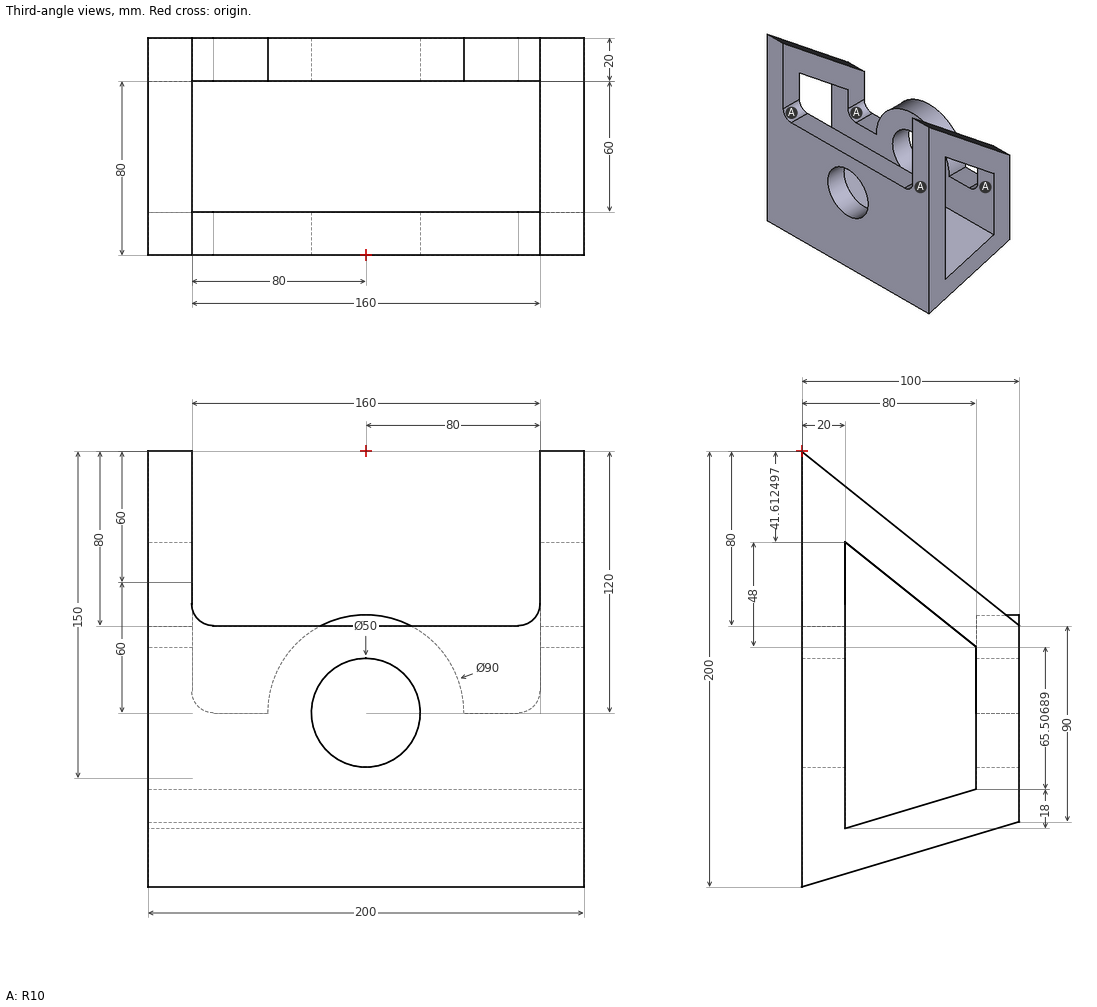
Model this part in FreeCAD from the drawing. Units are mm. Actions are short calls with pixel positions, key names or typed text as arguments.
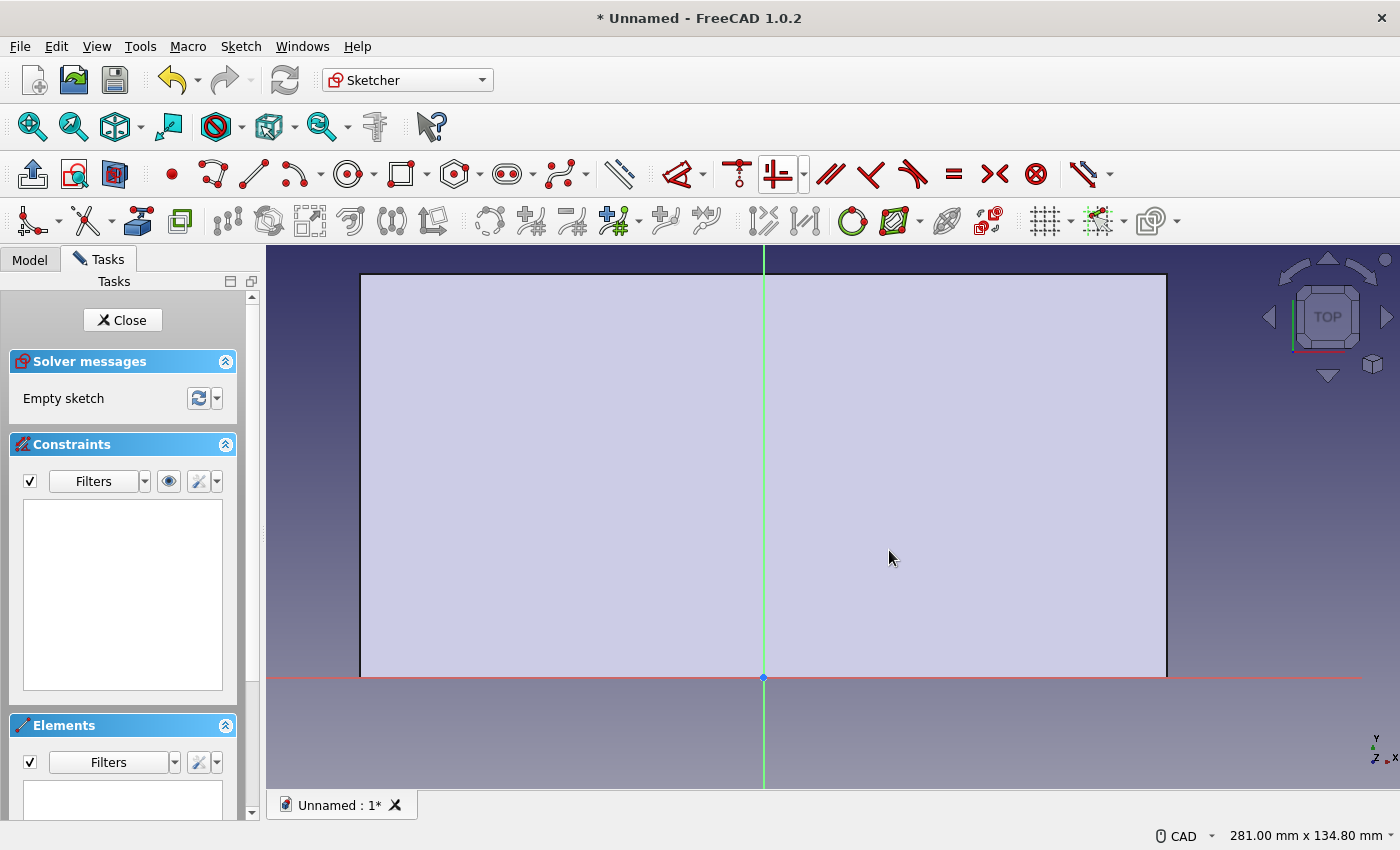
click(400, 174)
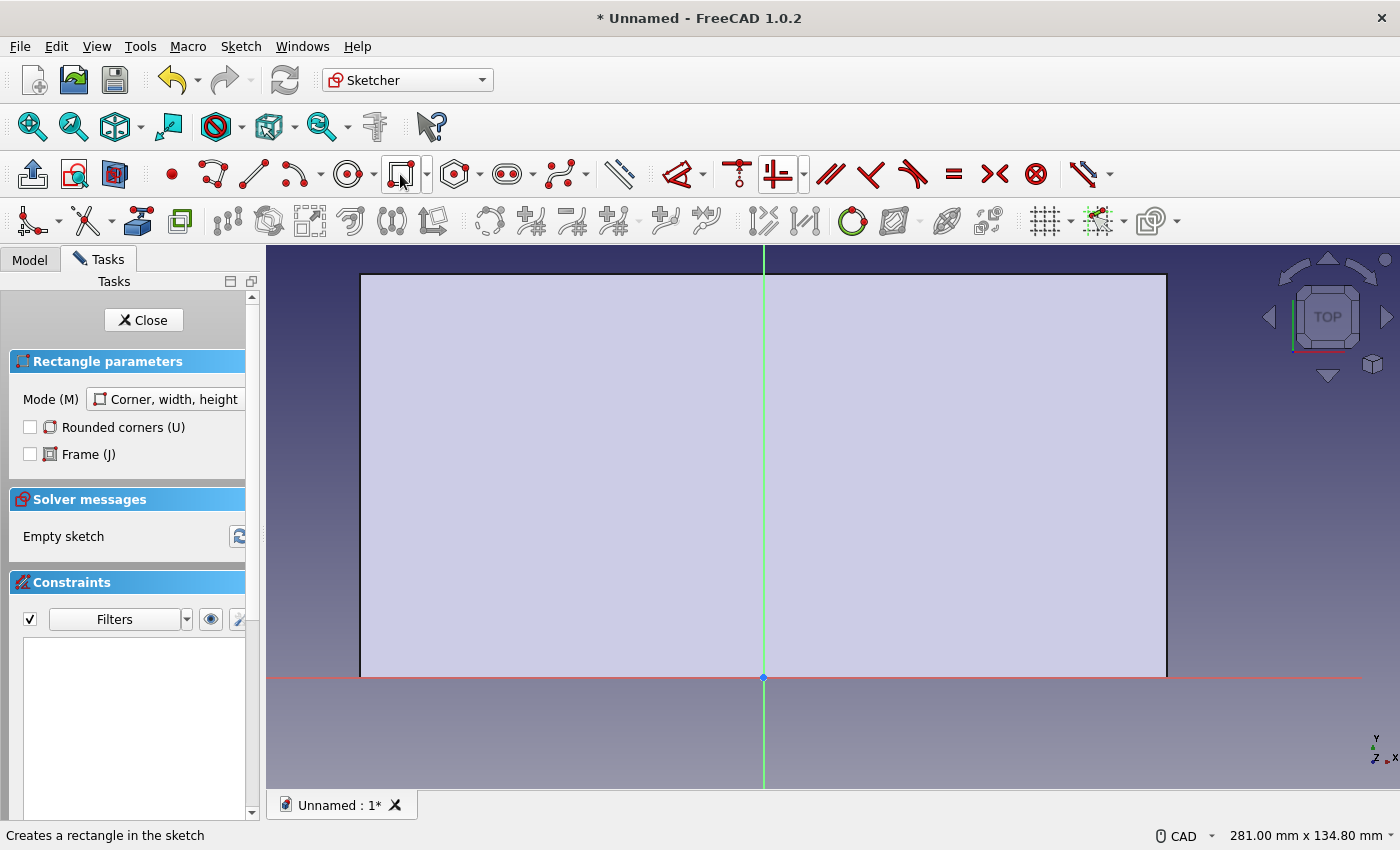
click(441, 355)
move(1087, 597)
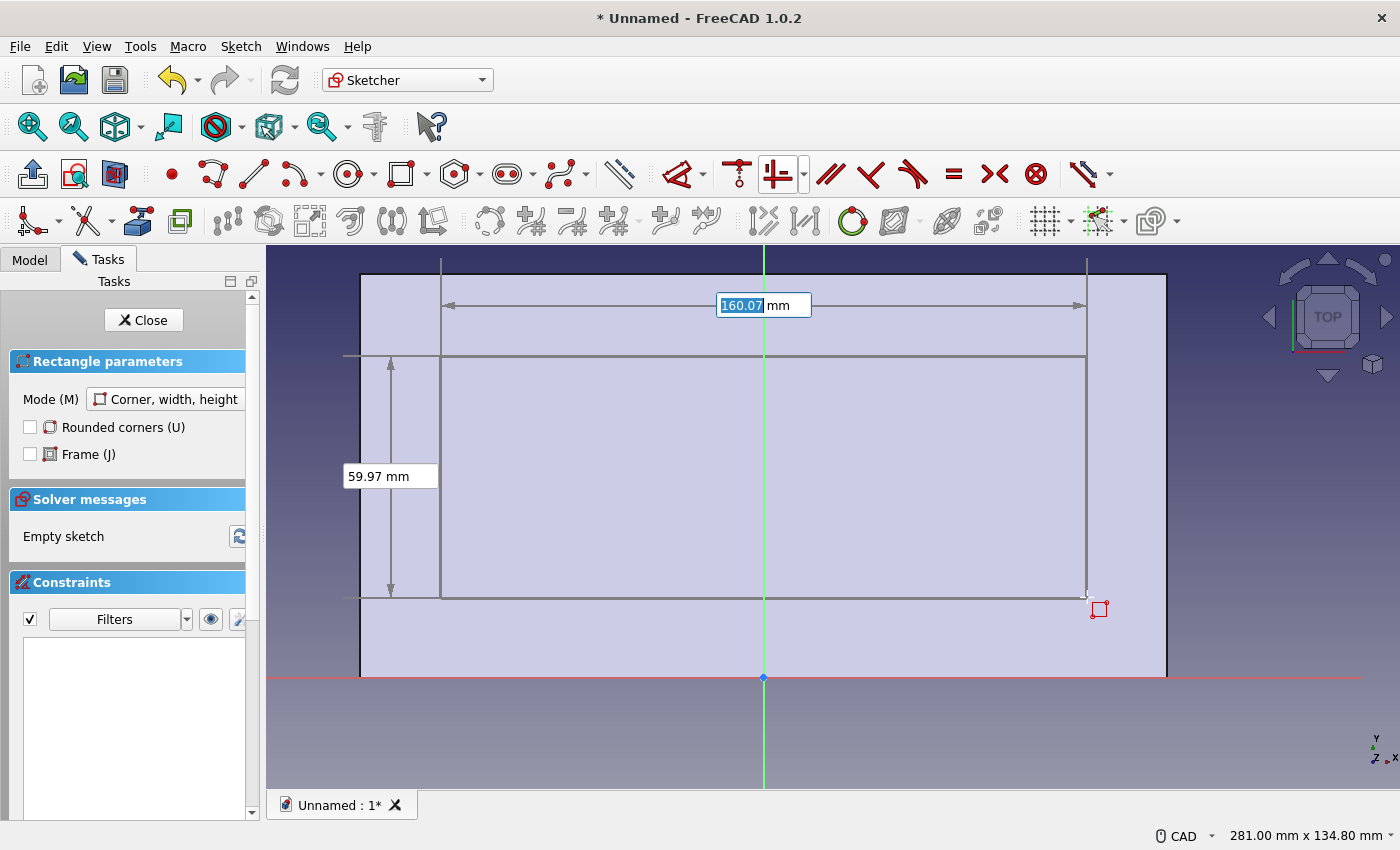
text(160)
key(Tab)
text(60)
key(Return)
key(Escape)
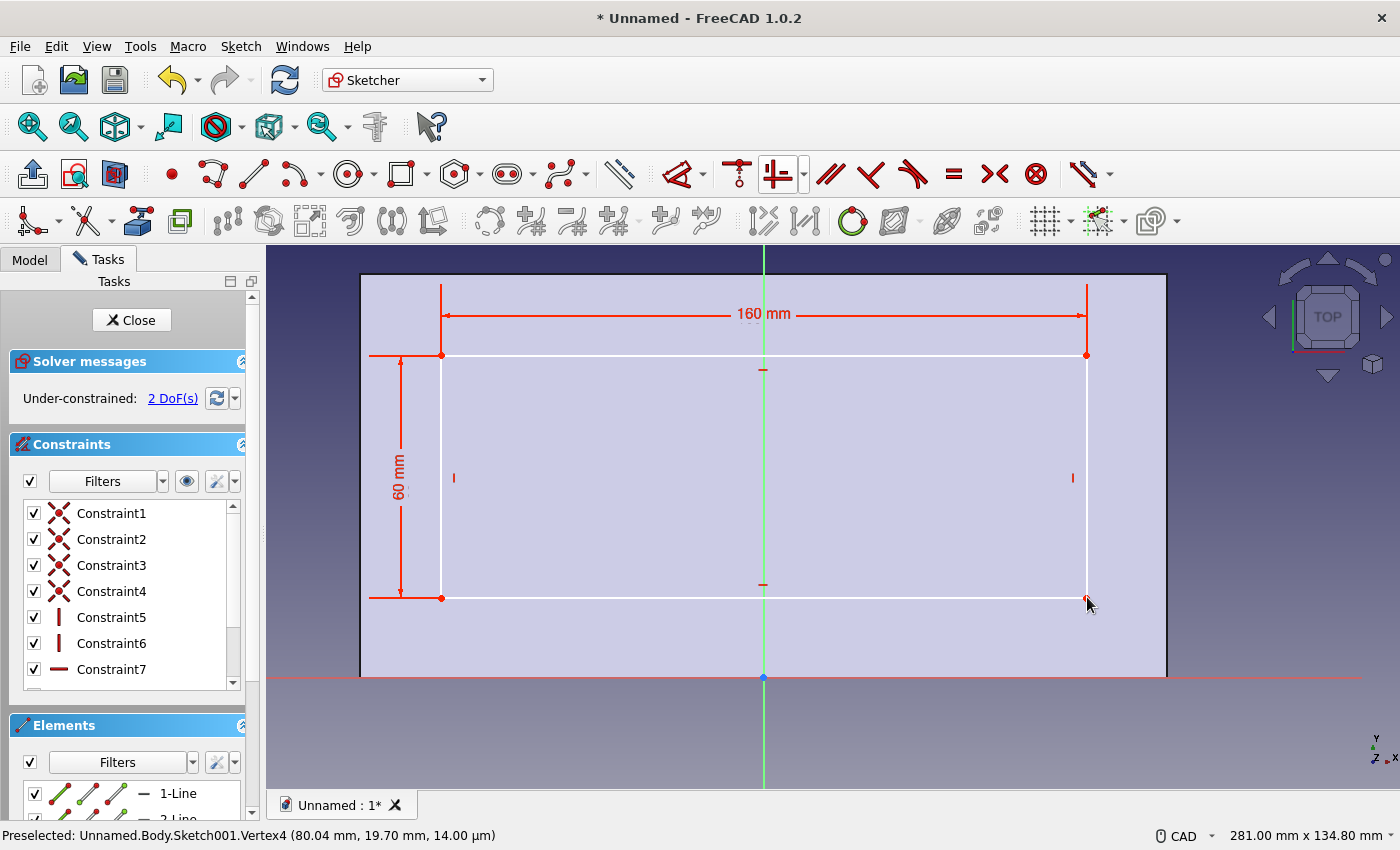
key(d)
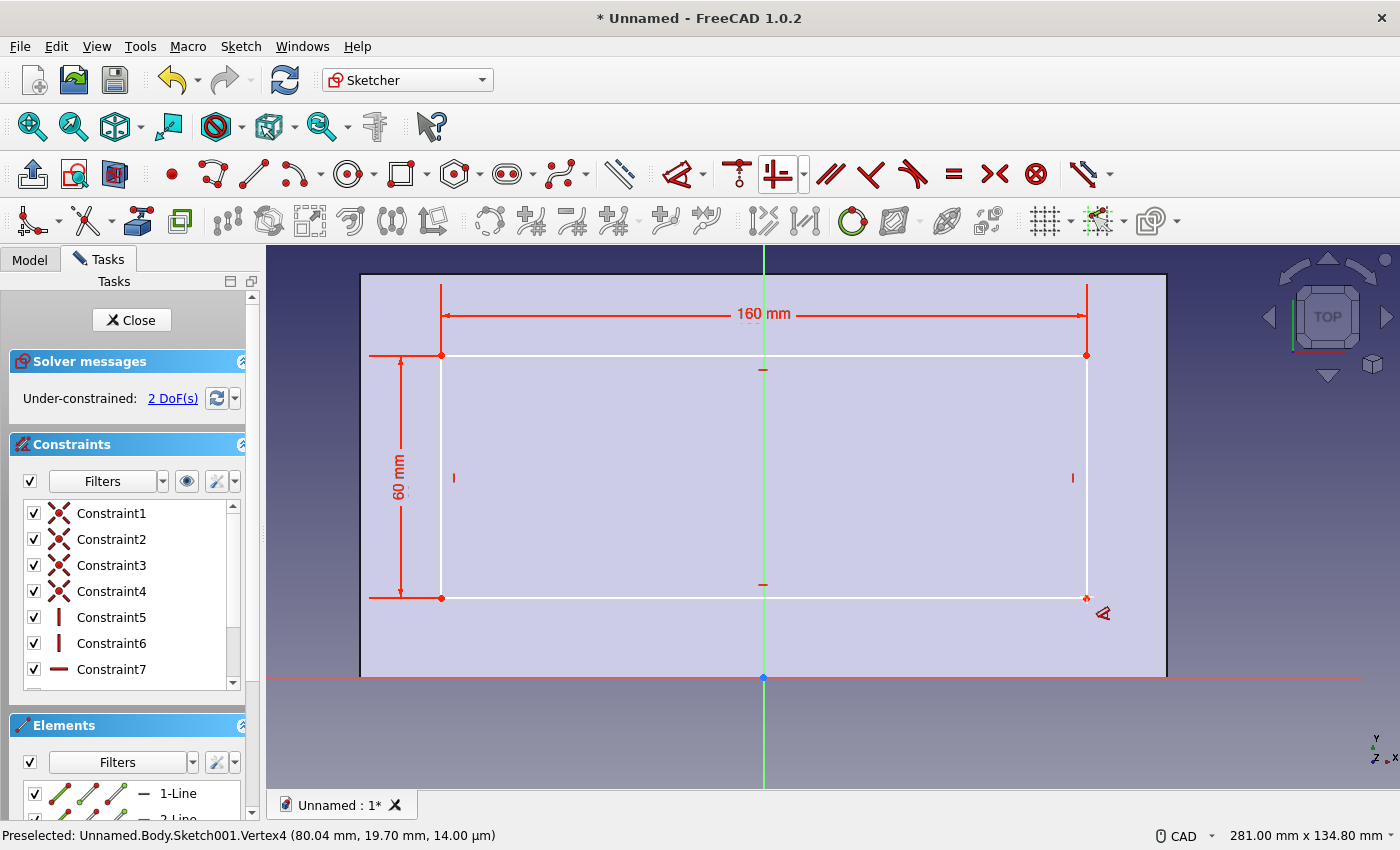
click(441, 356)
click(602, 712)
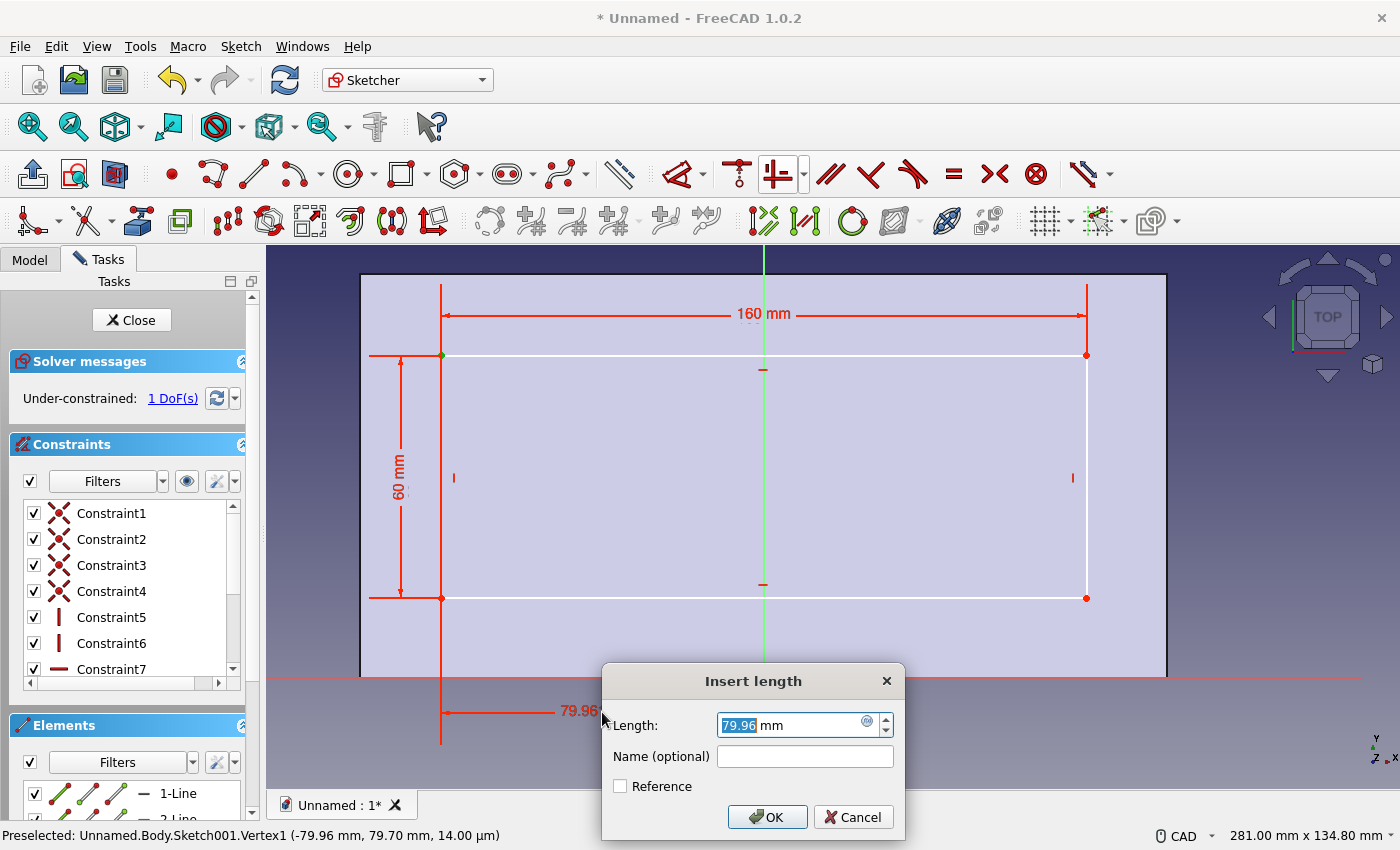
text(80)
key(Return)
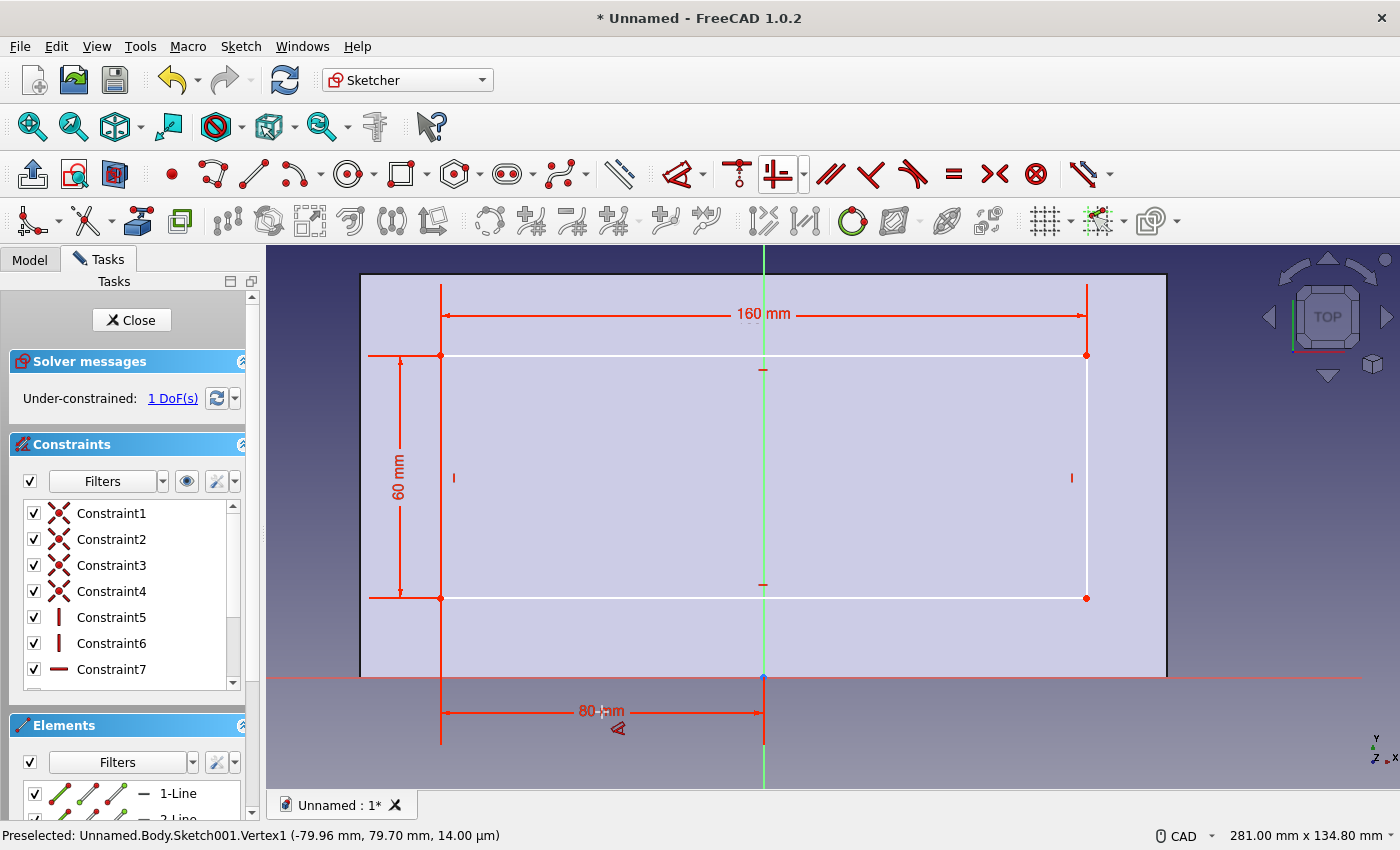
click(441, 356)
click(407, 517)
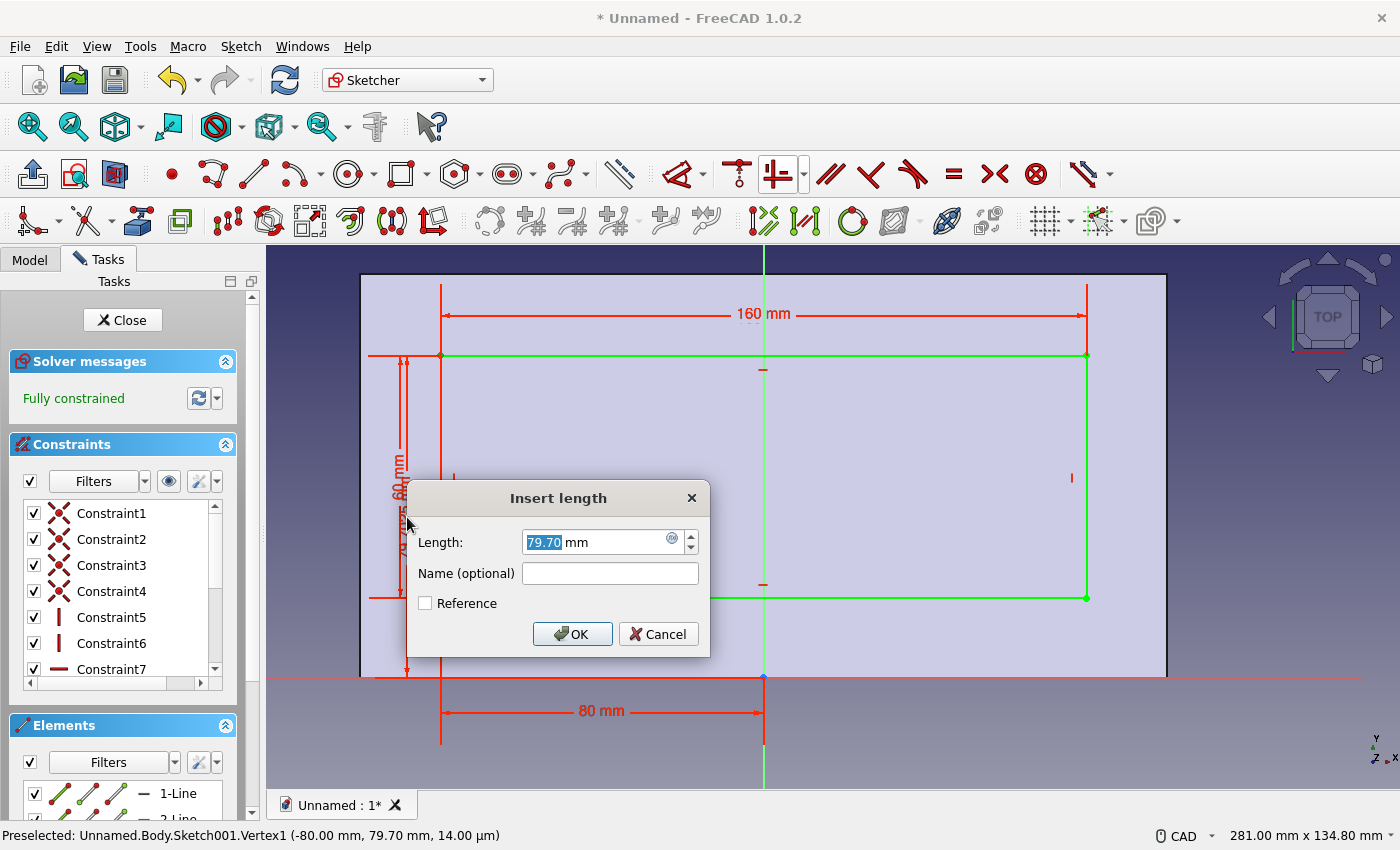
text(80)
key(Return)
key(Escape)